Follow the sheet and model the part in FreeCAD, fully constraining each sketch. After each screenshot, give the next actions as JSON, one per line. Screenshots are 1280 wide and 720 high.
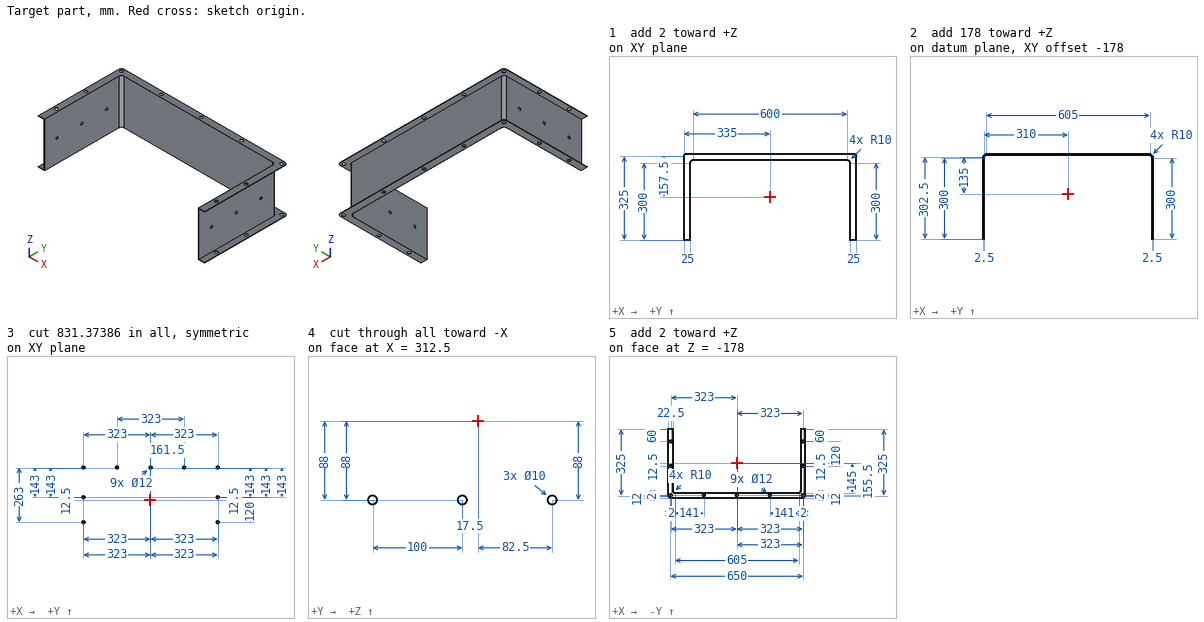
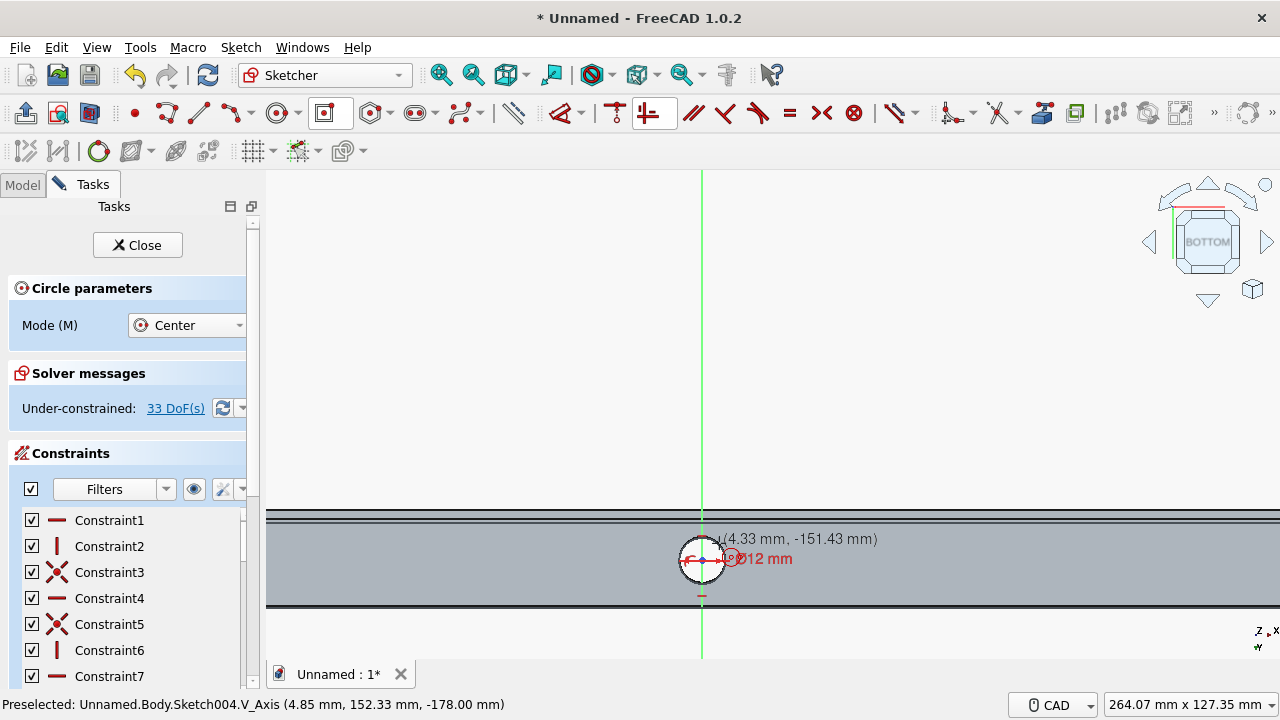
{"action": "scroll", "coordinate": [705, 562], "scroll_direction": "down", "scroll_amount": 7}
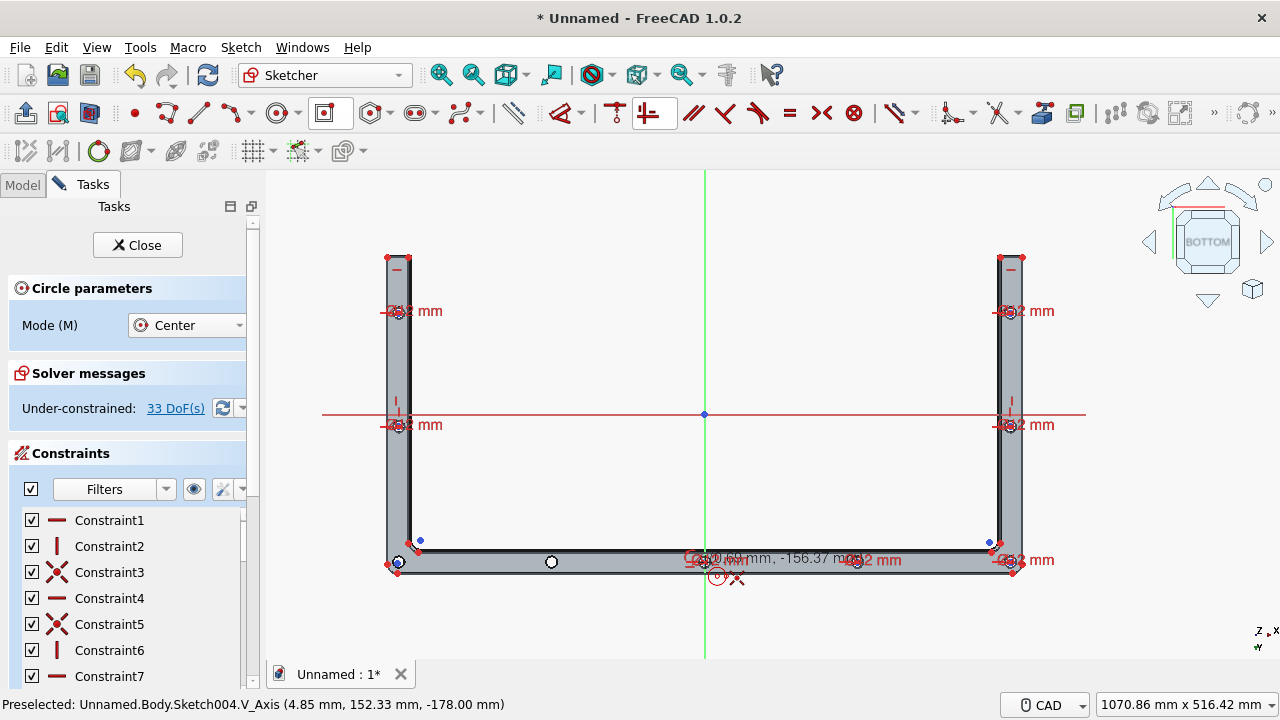
{"action": "scroll", "coordinate": [552, 562], "scroll_direction": "up", "scroll_amount": 7}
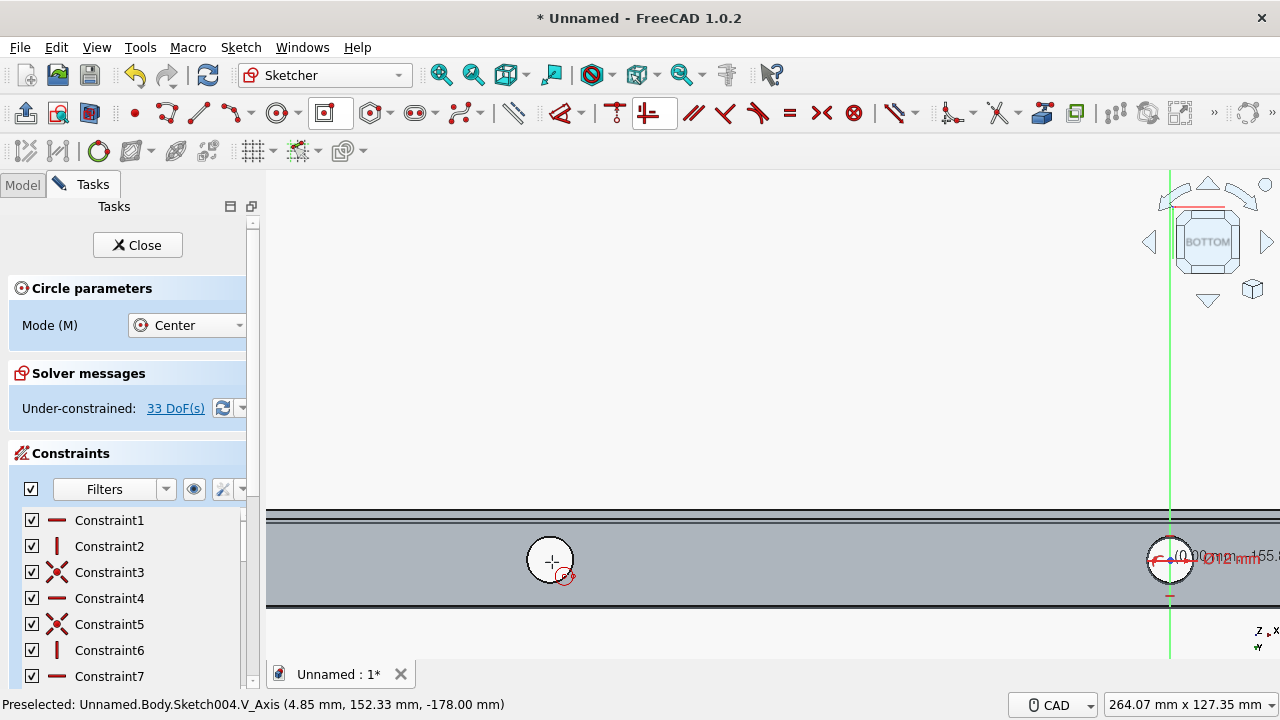
{"action": "left_click", "coordinate": [550, 560]}
{"action": "mouse_move", "coordinate": [566, 543]}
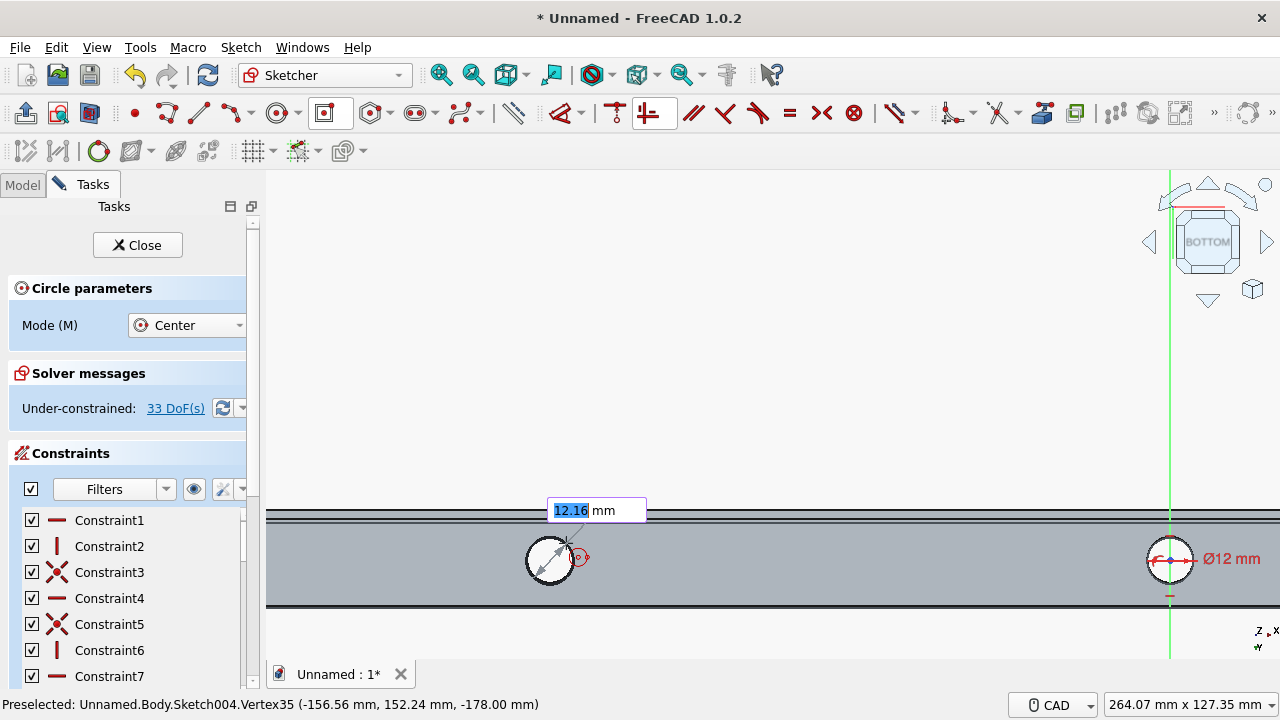
{"action": "type", "text": "12"}
{"action": "key", "text": "Return"}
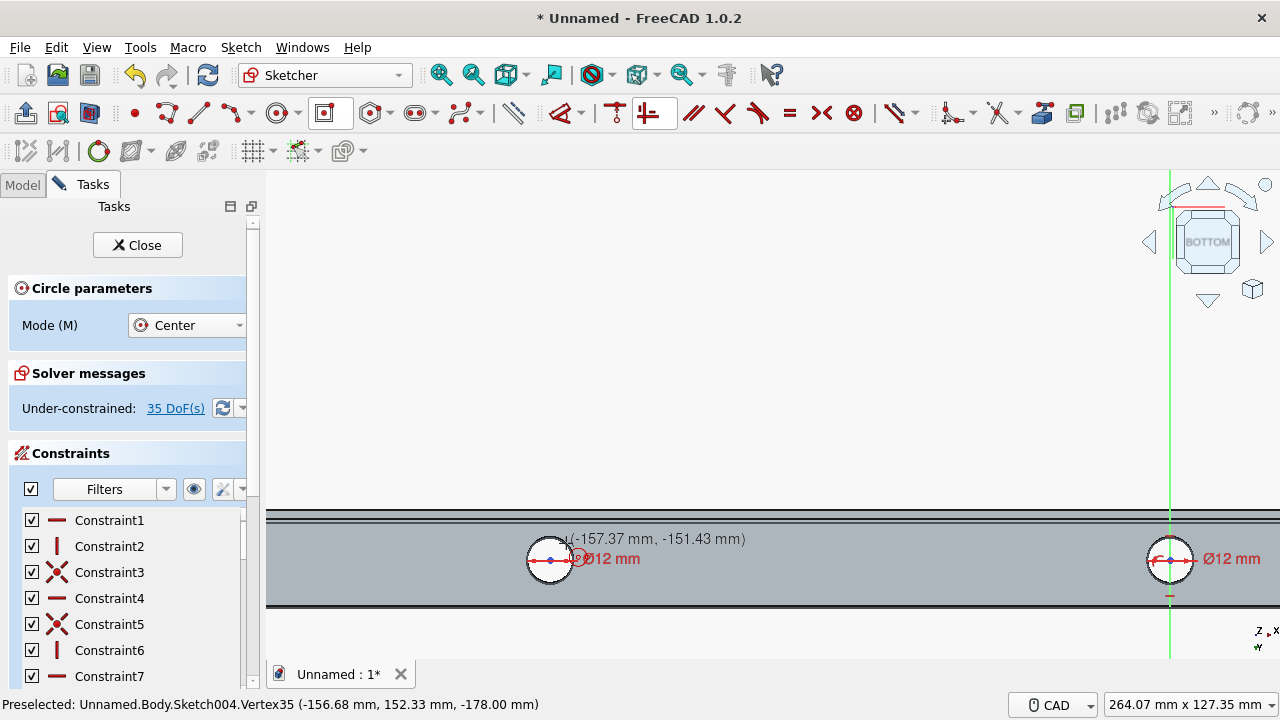
{"action": "scroll", "coordinate": [552, 562], "scroll_direction": "down", "scroll_amount": 7}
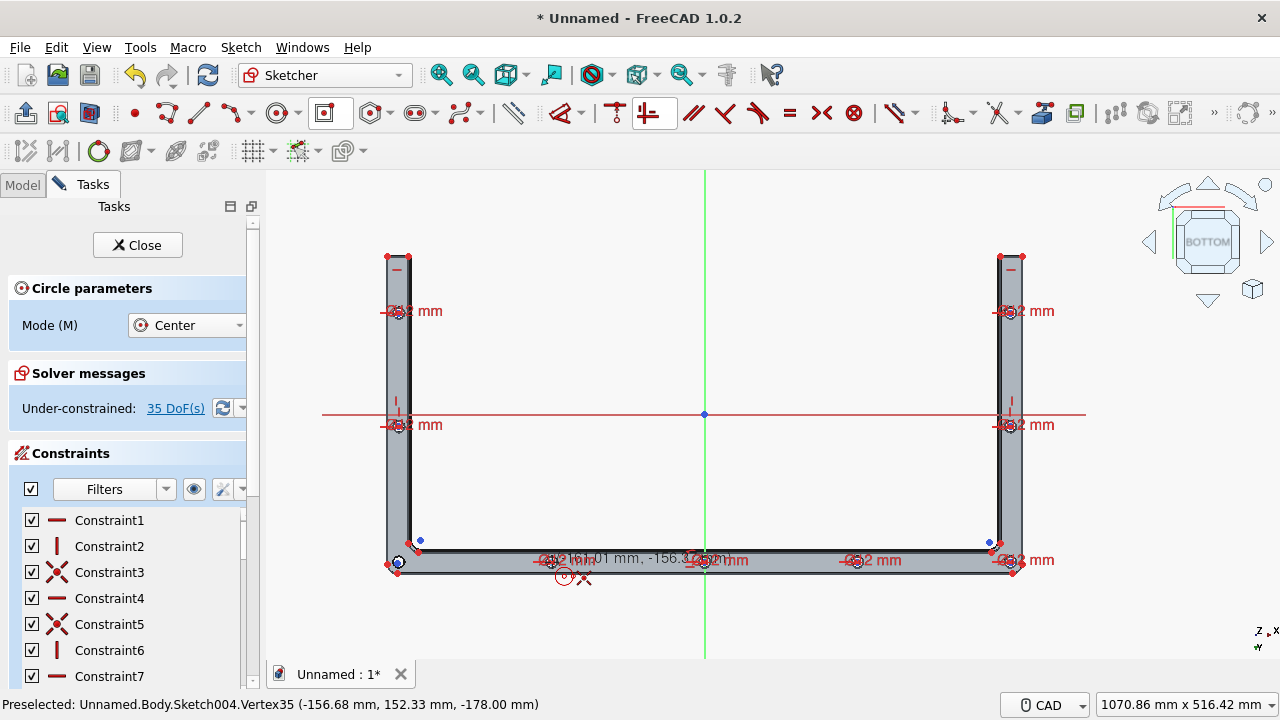
{"action": "scroll", "coordinate": [399, 562], "scroll_direction": "up", "scroll_amount": 9}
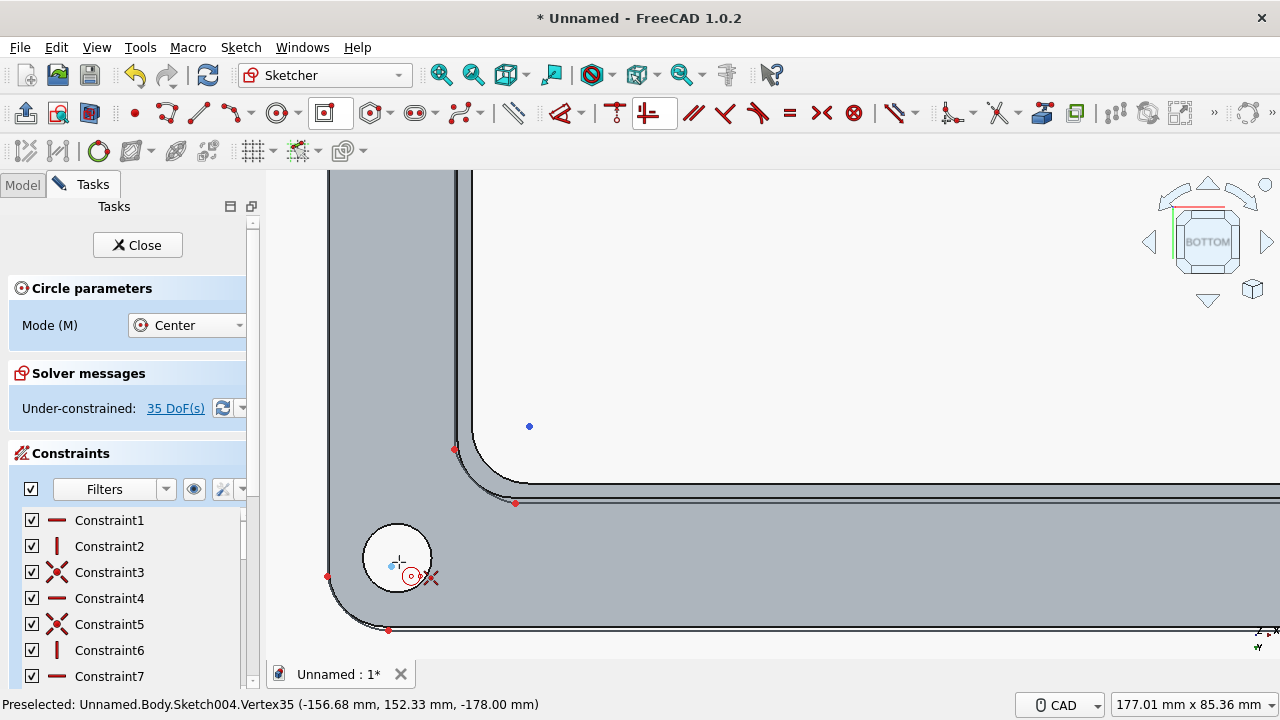
{"action": "left_click", "coordinate": [397, 558]}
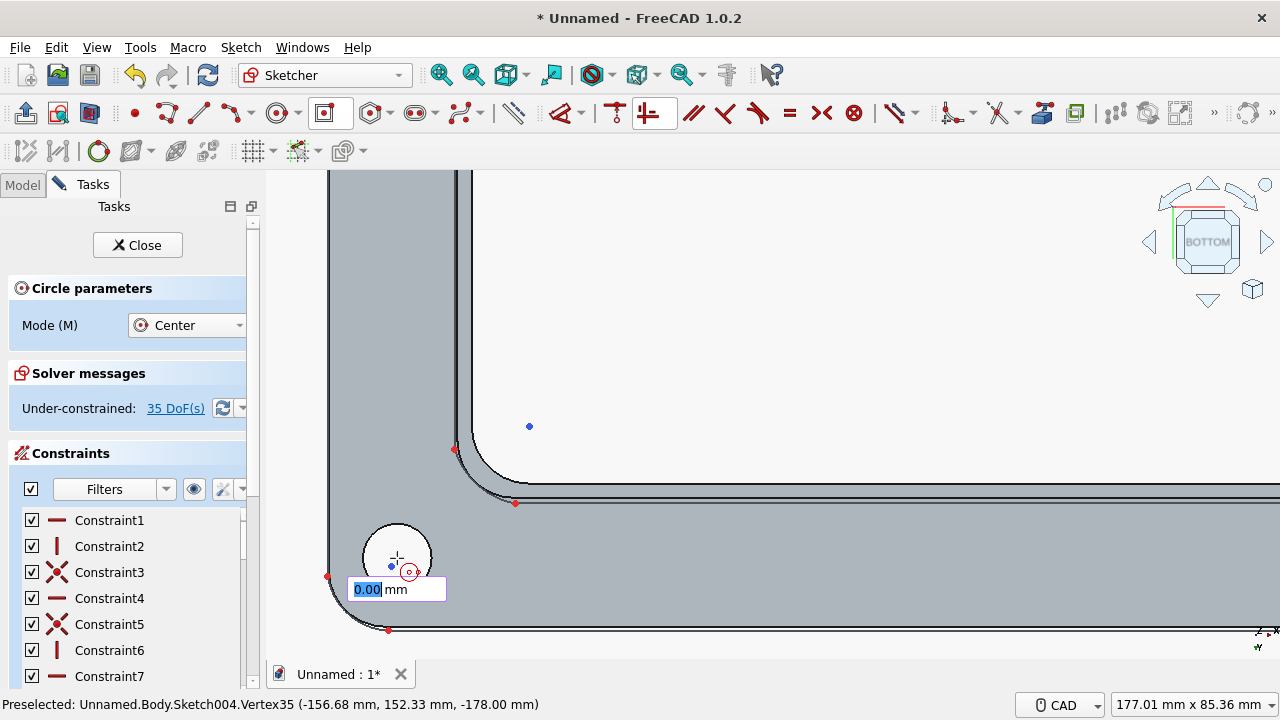
{"action": "scroll", "coordinate": [399, 562], "scroll_direction": "down", "scroll_amount": 9}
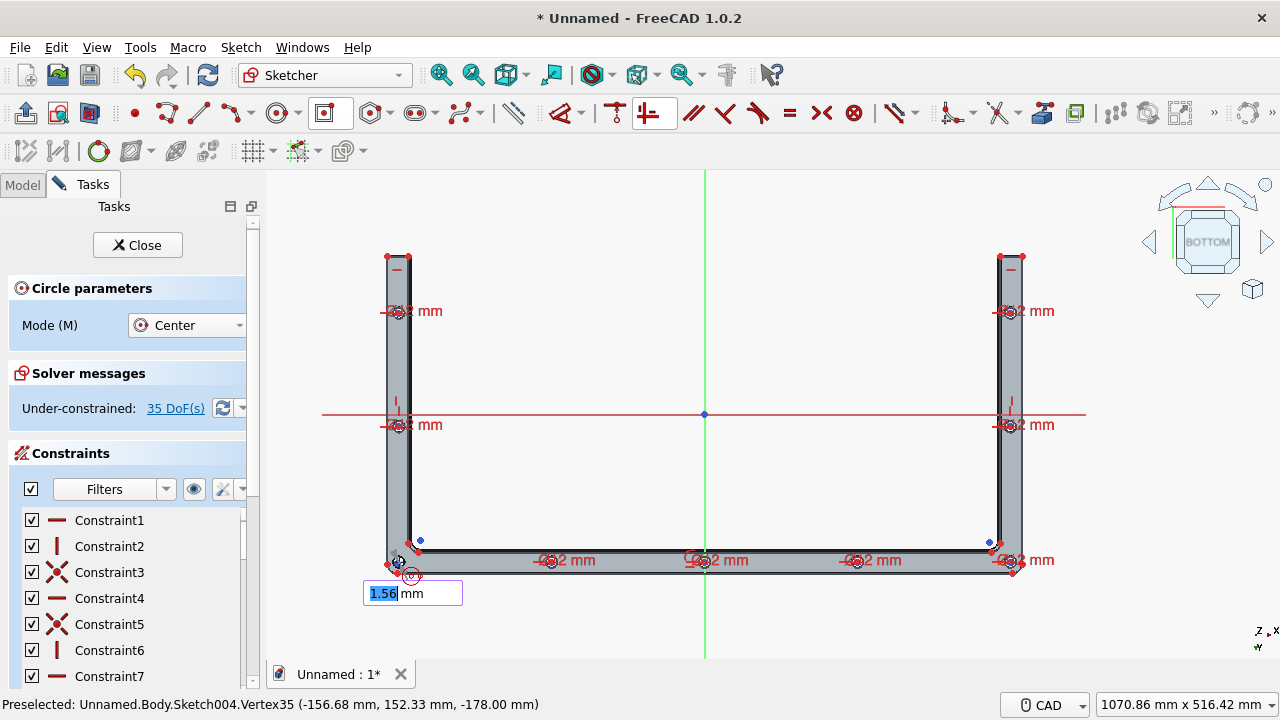
{"action": "scroll", "coordinate": [403, 558], "scroll_direction": "up", "scroll_amount": 4}
{"action": "mouse_move", "coordinate": [402, 557]}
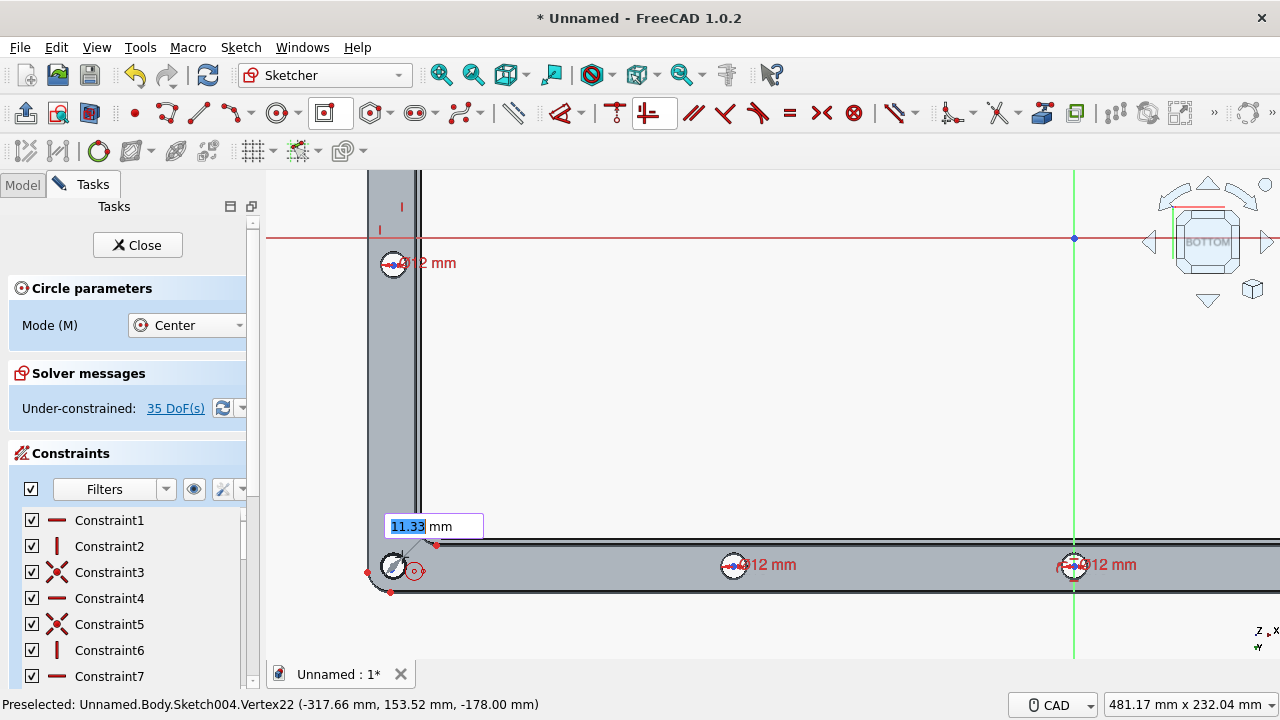
{"action": "type", "text": "12"}
{"action": "key", "text": "Return"}
{"action": "key", "text": "Escape"}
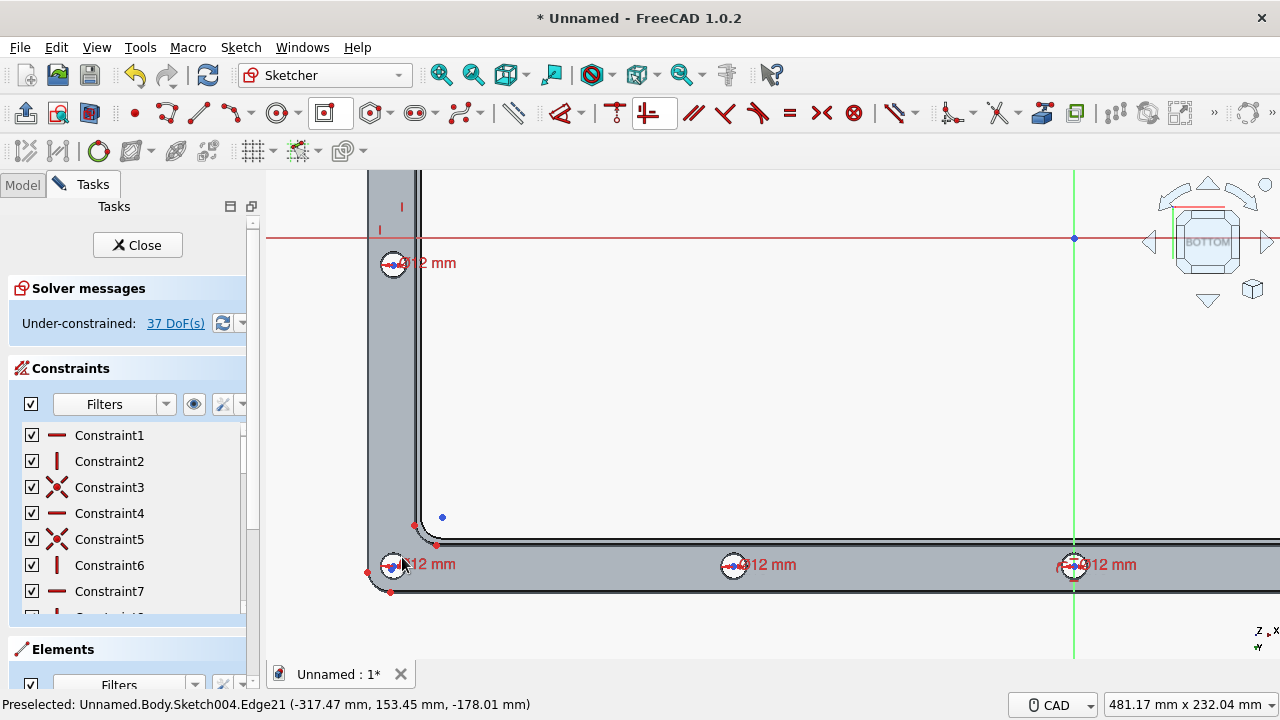
{"action": "left_click", "coordinate": [820, 546]}